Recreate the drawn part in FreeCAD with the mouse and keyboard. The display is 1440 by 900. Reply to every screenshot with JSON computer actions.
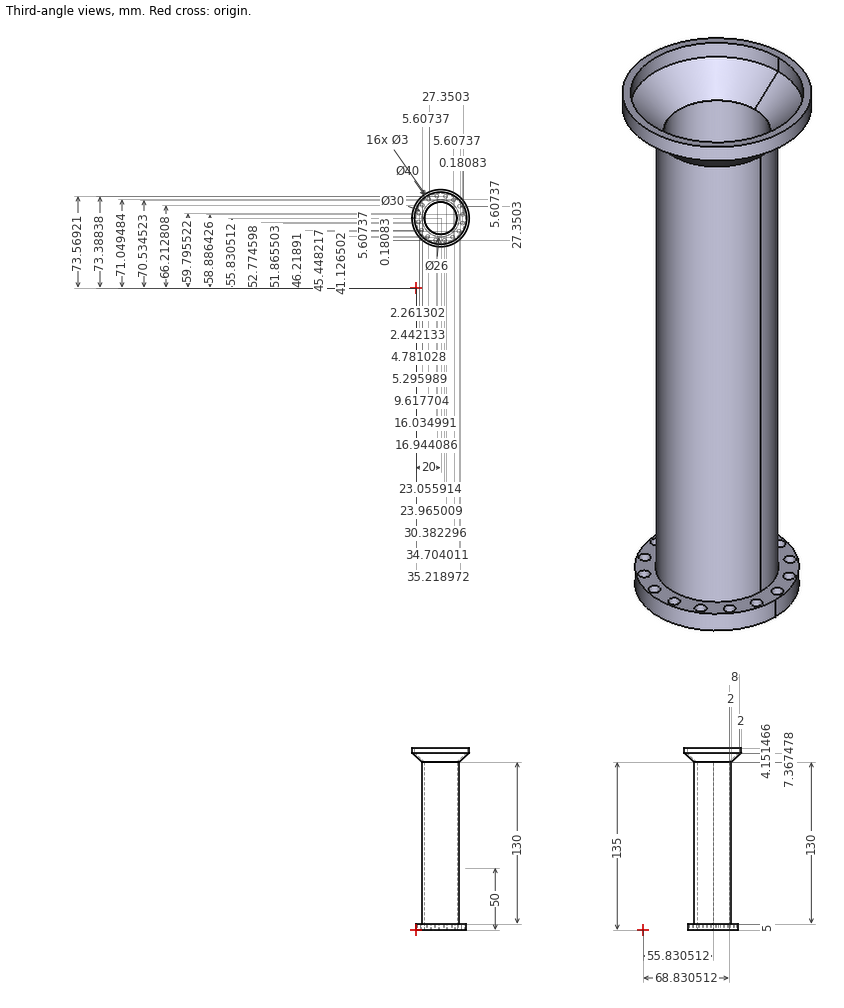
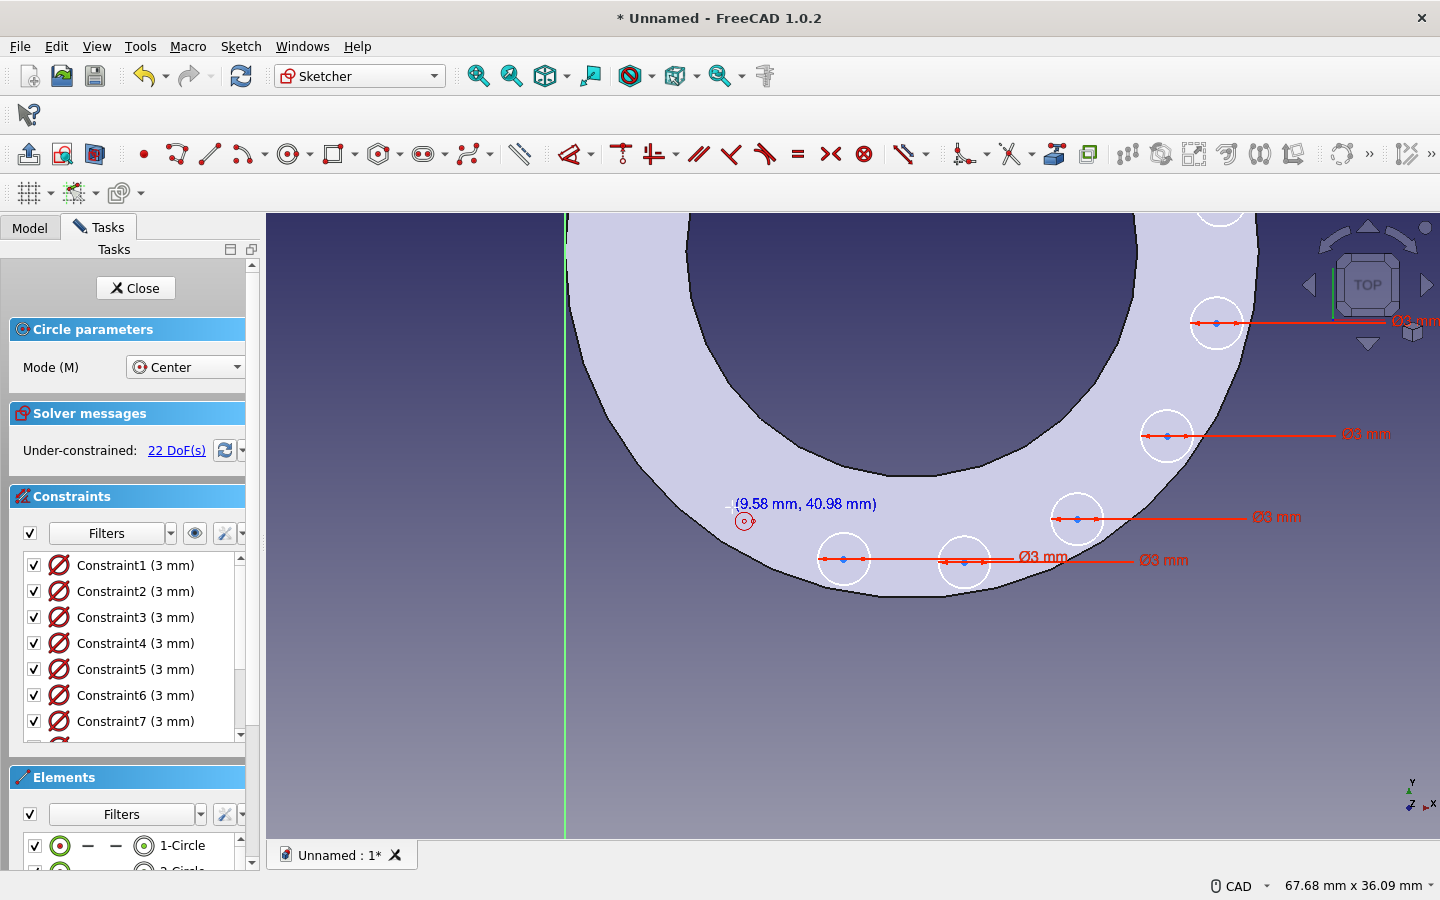
{"action": "scroll", "coordinate": [732, 507], "scroll_direction": "down", "scroll_amount": 6}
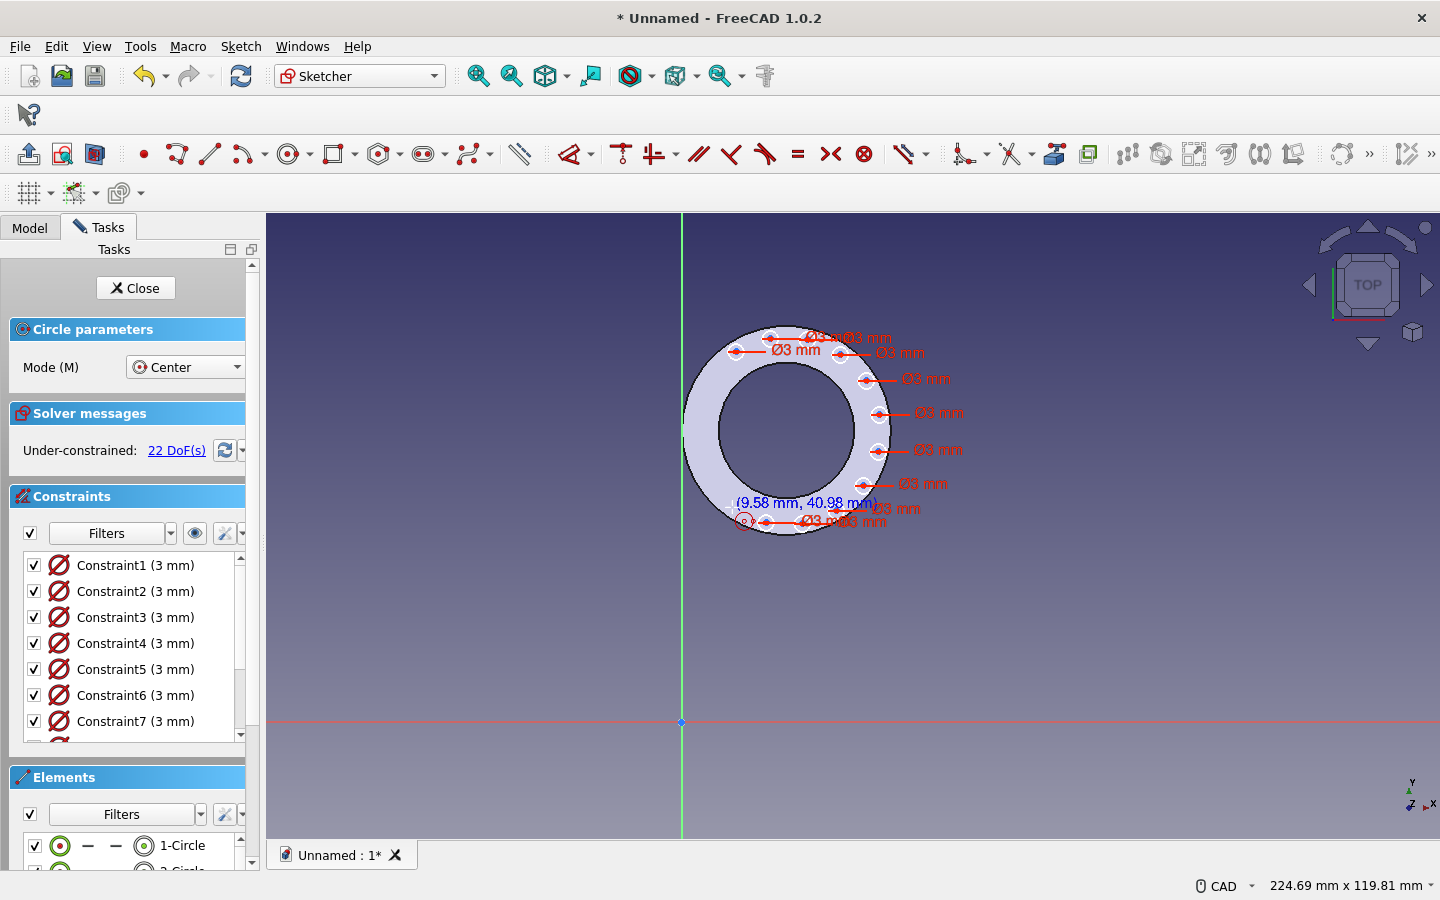
{"action": "left_click", "coordinate": [732, 507]}
{"action": "mouse_move", "coordinate": [738, 502]}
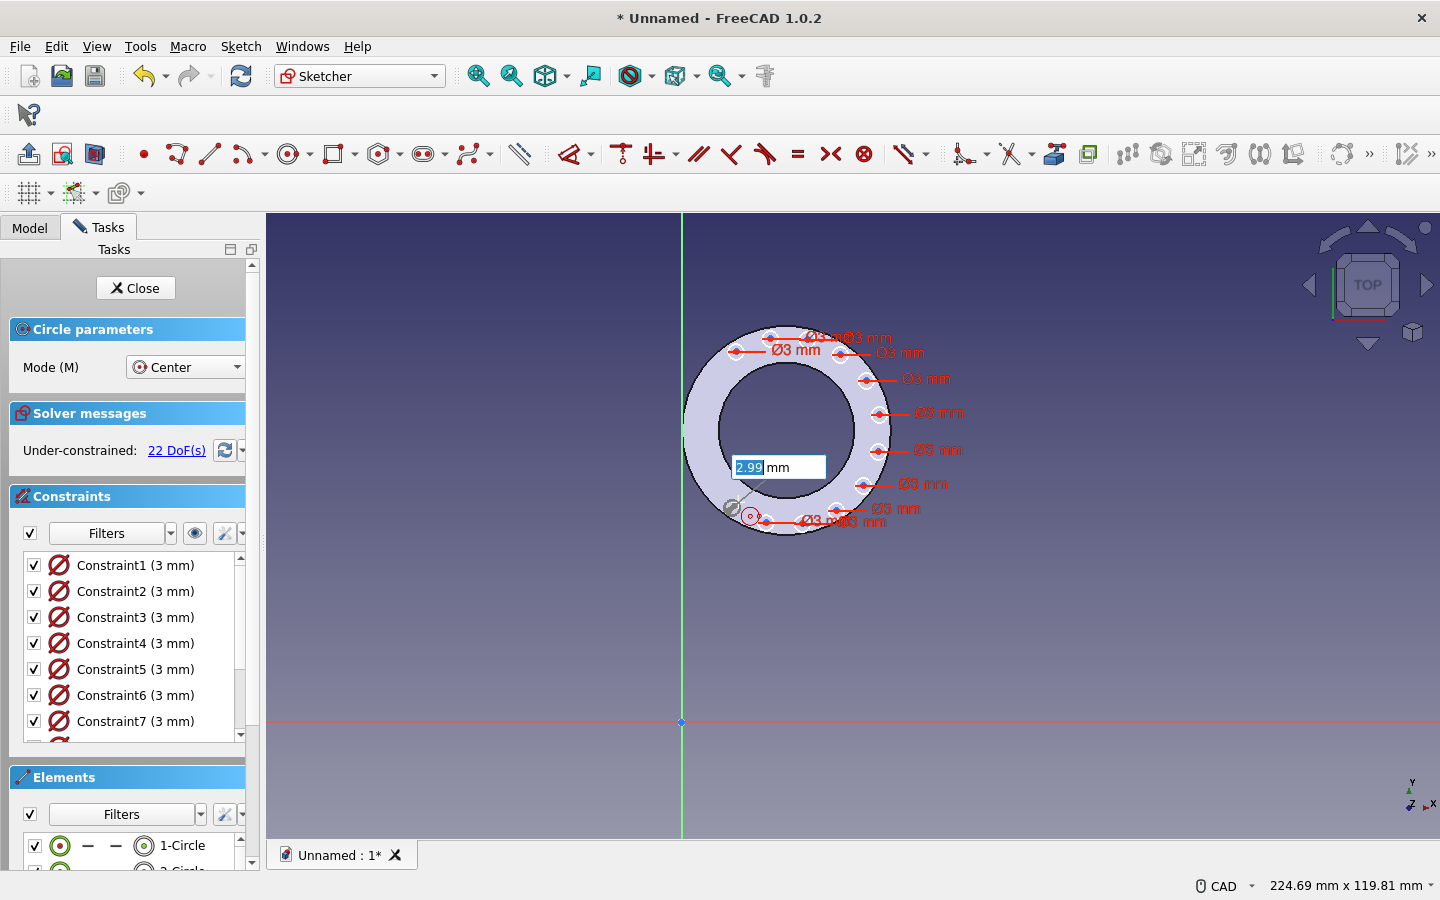
{"action": "type", "text": "3"}
{"action": "key", "text": "Return"}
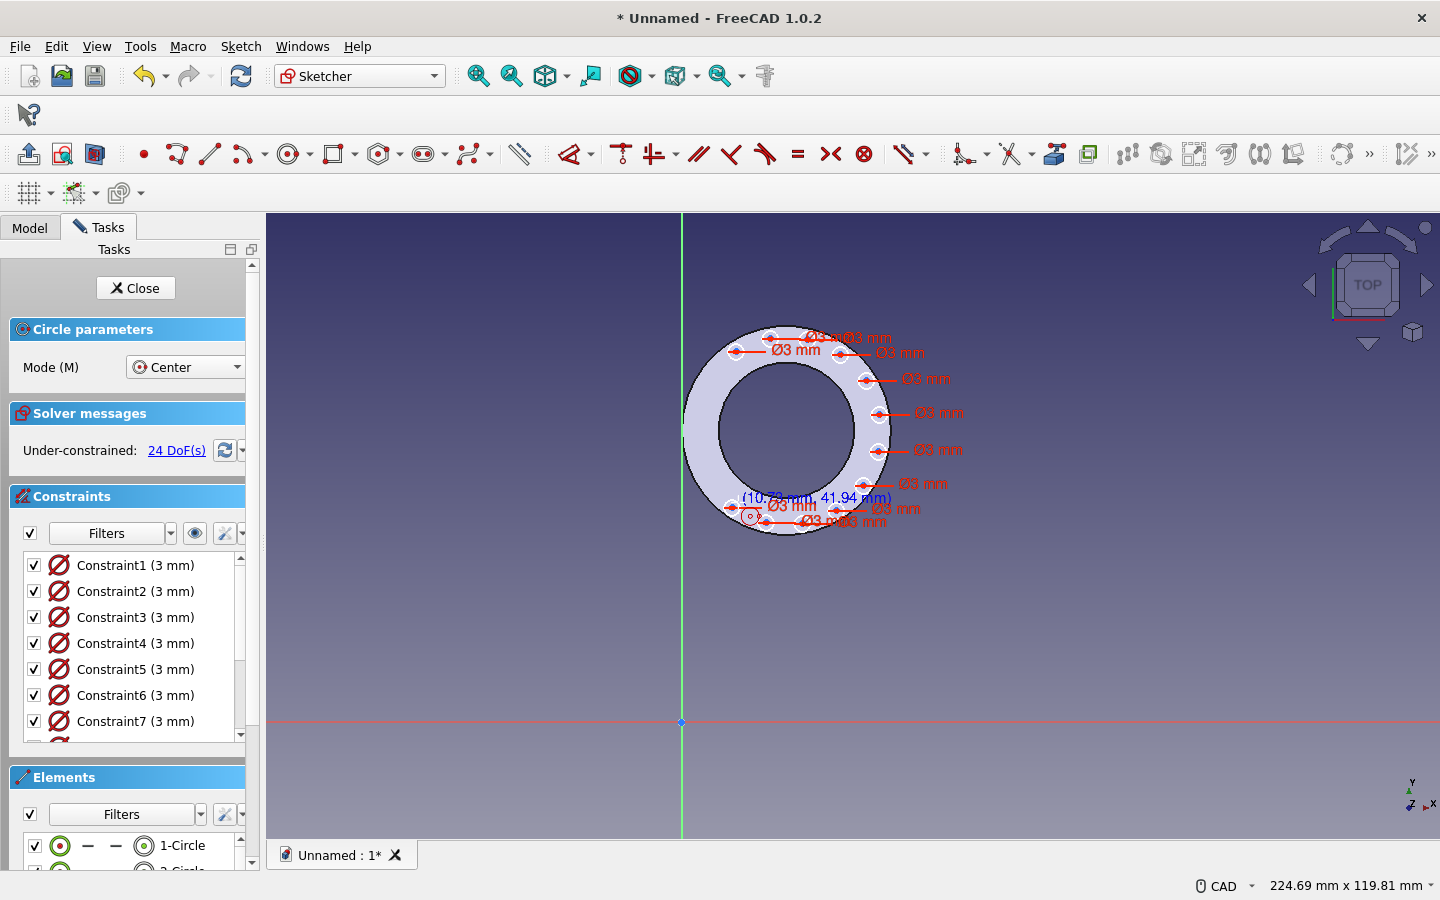
{"action": "scroll", "coordinate": [707, 481], "scroll_direction": "up", "scroll_amount": 6}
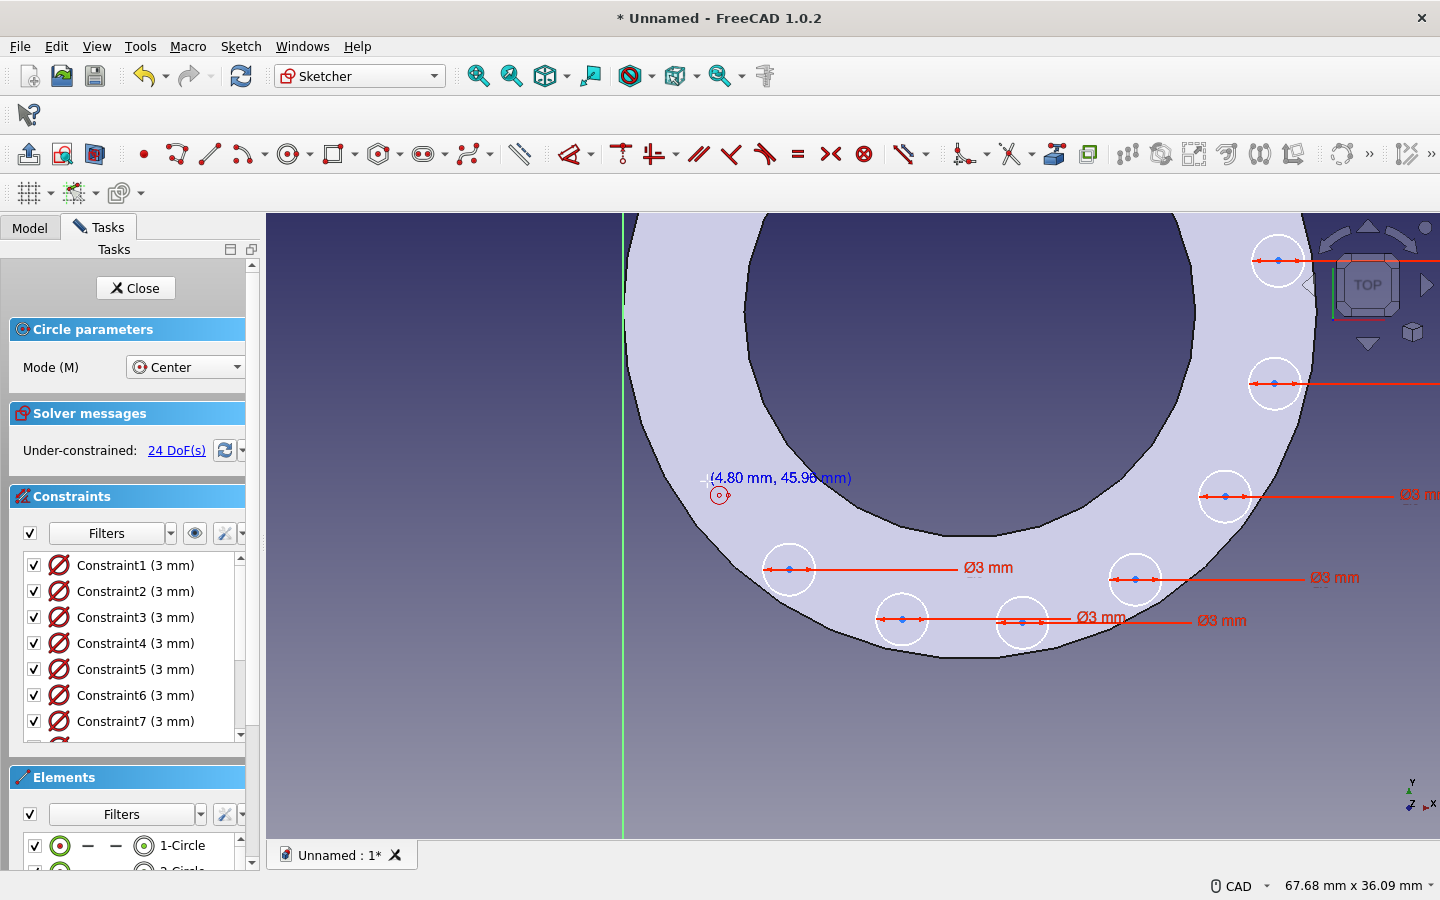
{"action": "scroll", "coordinate": [707, 481], "scroll_direction": "down", "scroll_amount": 6}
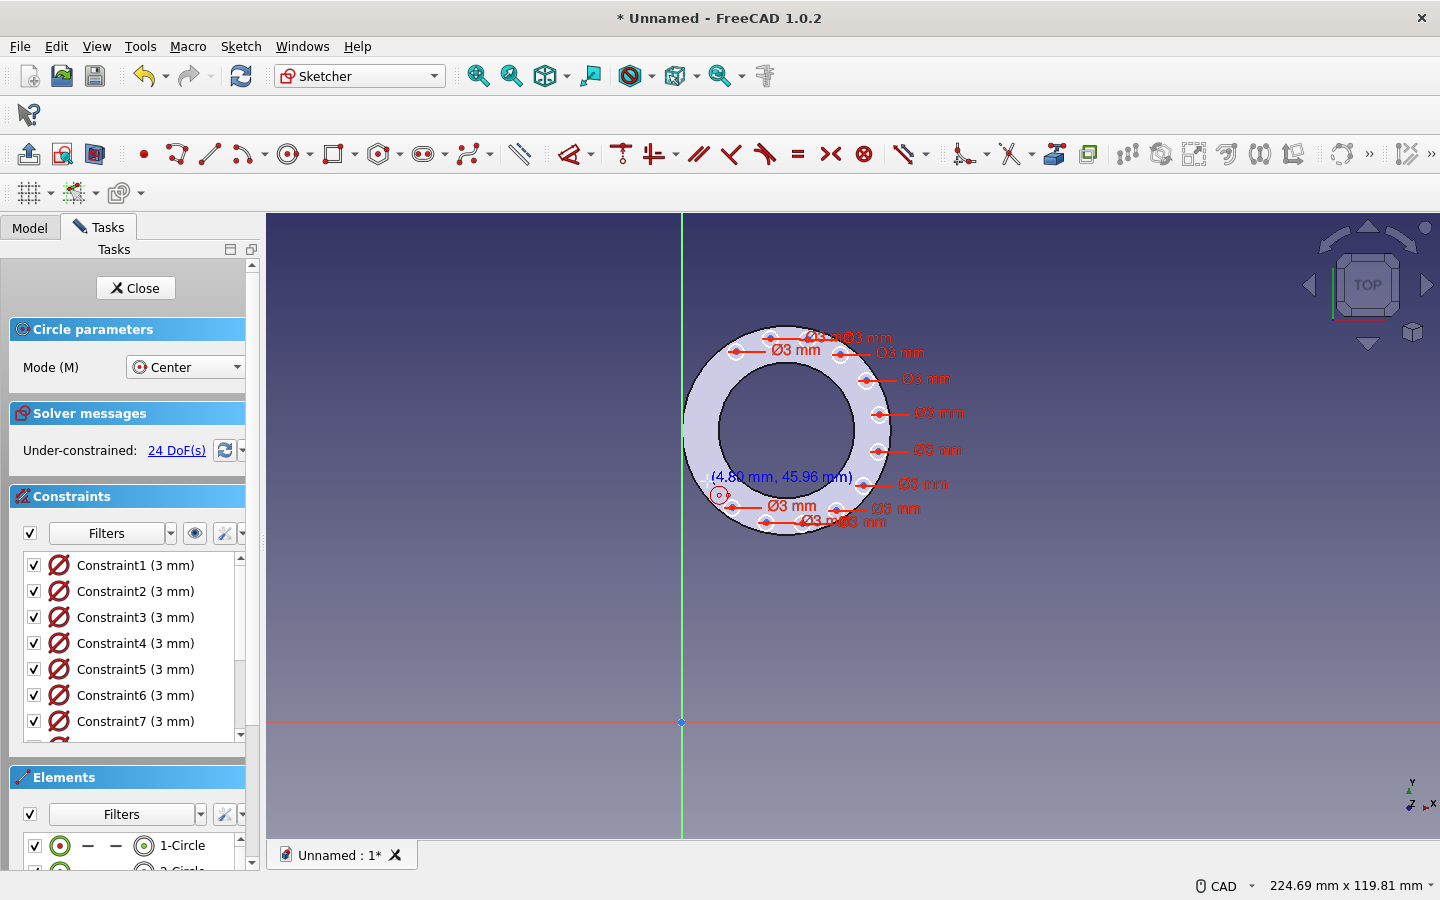
{"action": "left_click", "coordinate": [707, 481]}
{"action": "mouse_move", "coordinate": [712, 475]}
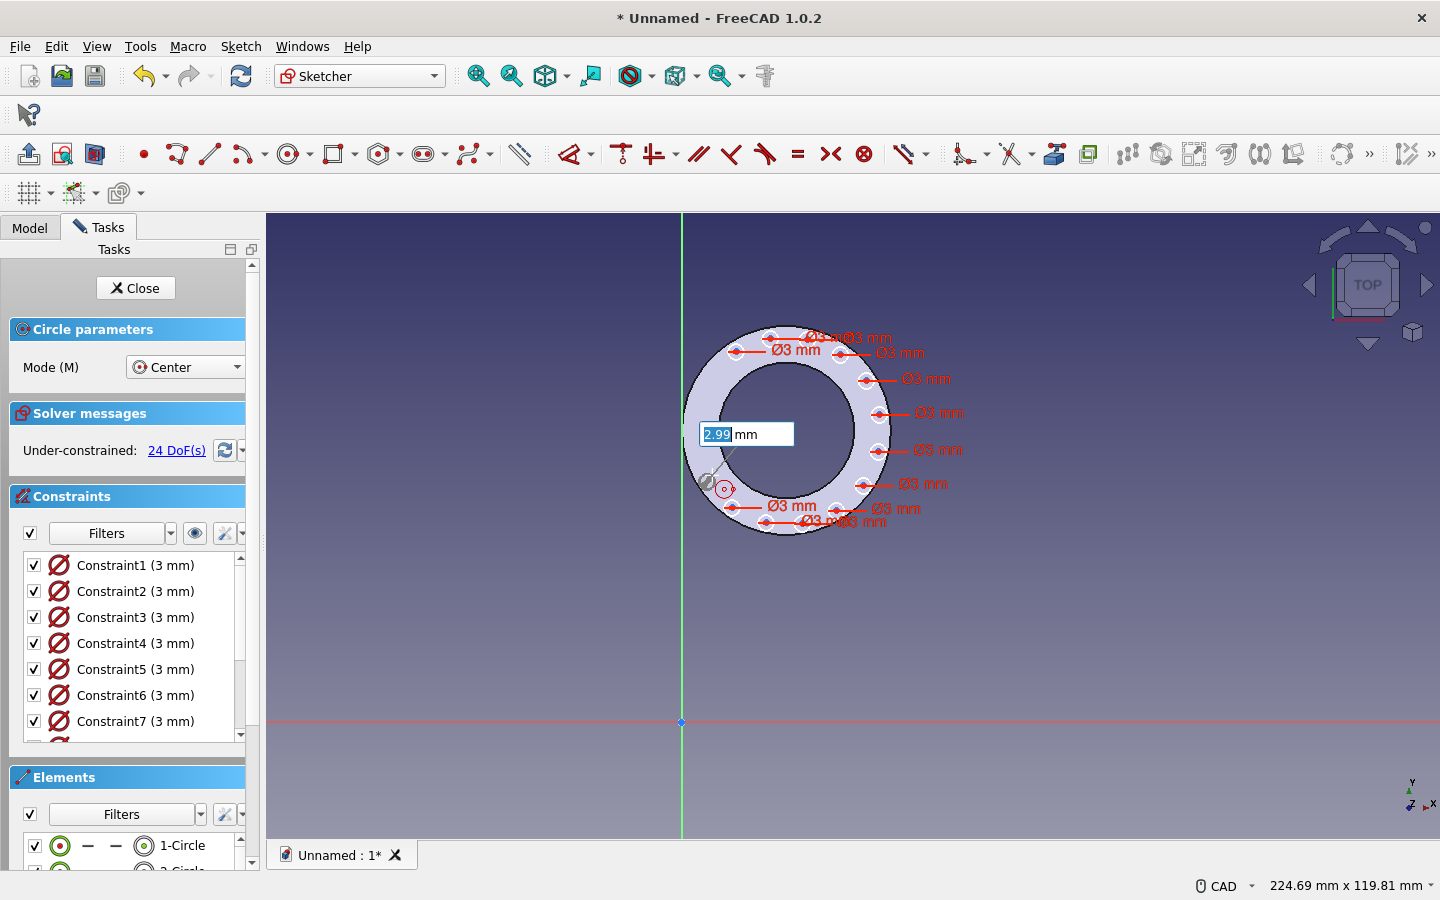
{"action": "type", "text": "3"}
{"action": "key", "text": "Return"}